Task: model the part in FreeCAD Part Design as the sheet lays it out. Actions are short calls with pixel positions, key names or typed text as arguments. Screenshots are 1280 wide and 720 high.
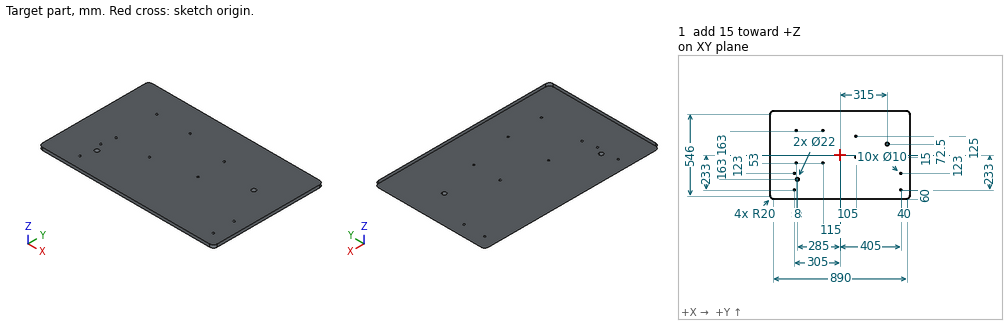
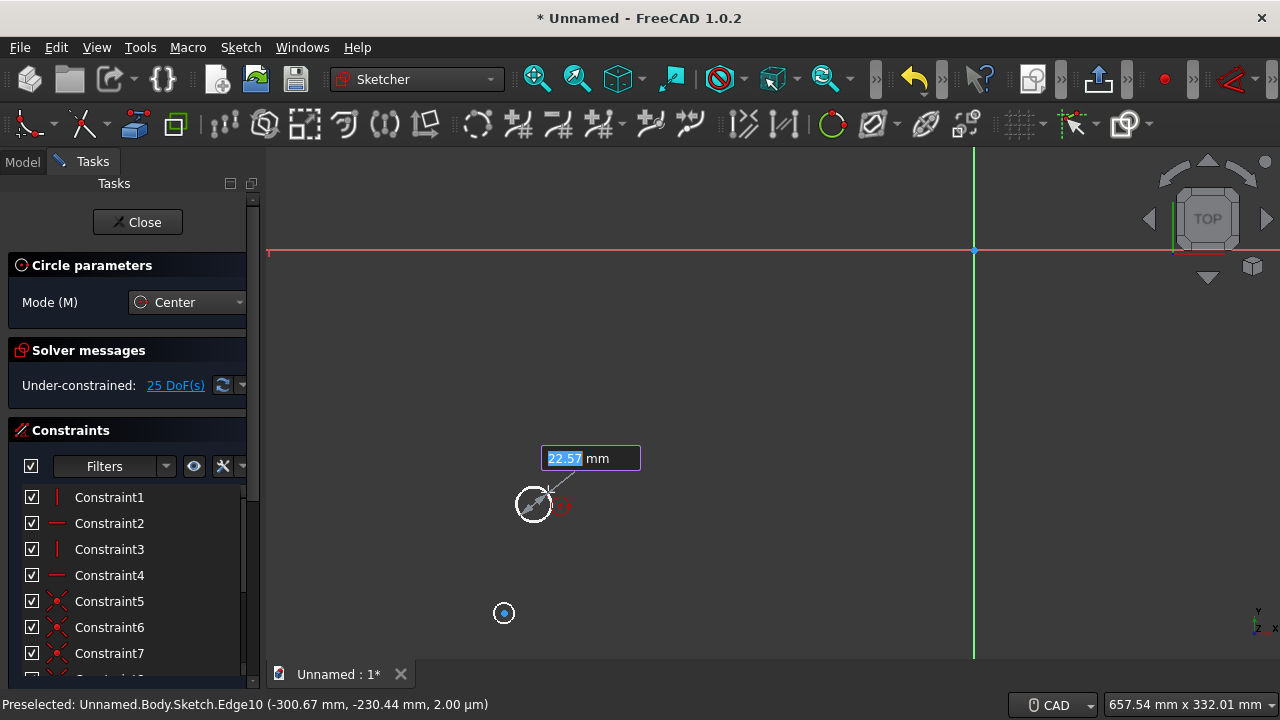
click(547, 489)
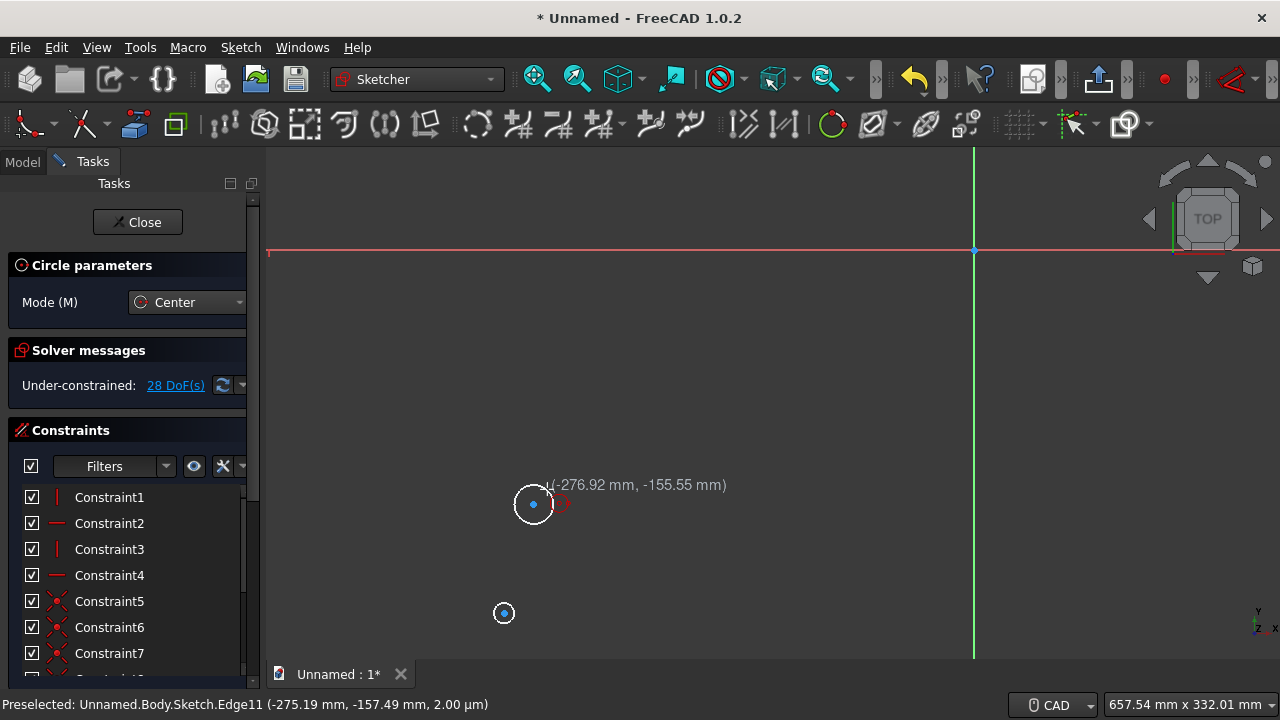
scroll(797, 332, up, 6)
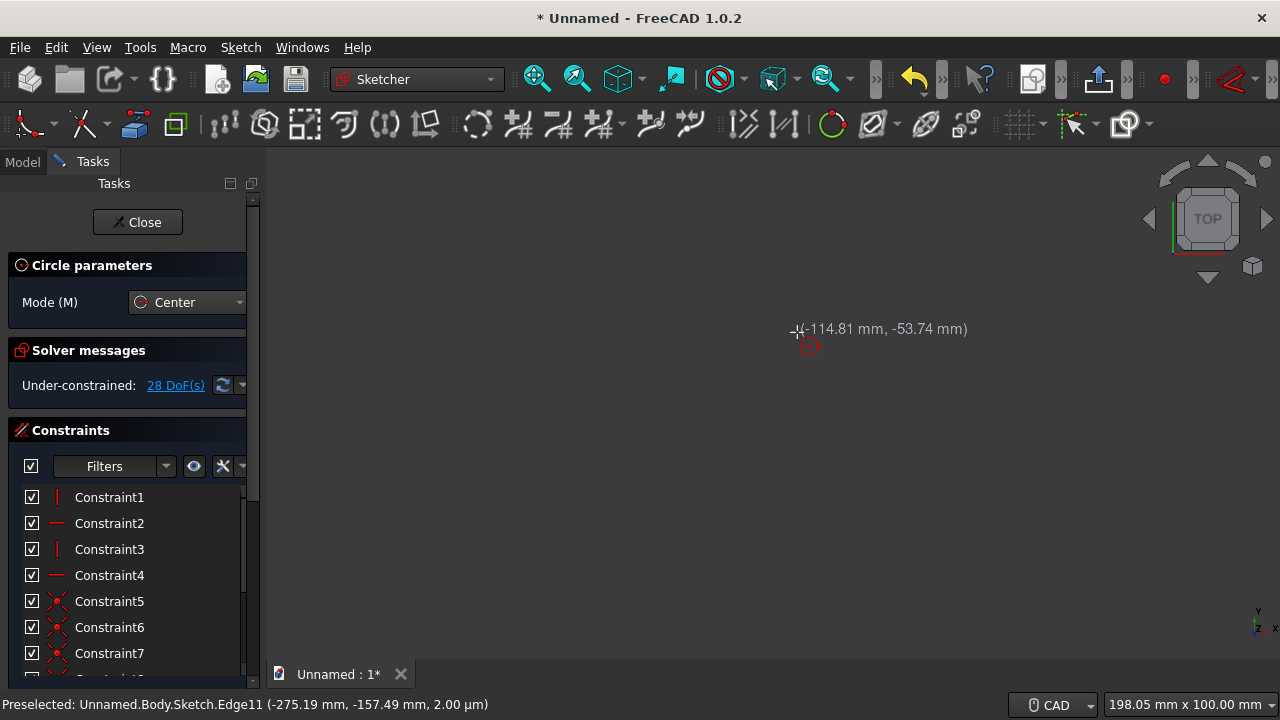
scroll(620, 446, down, 11)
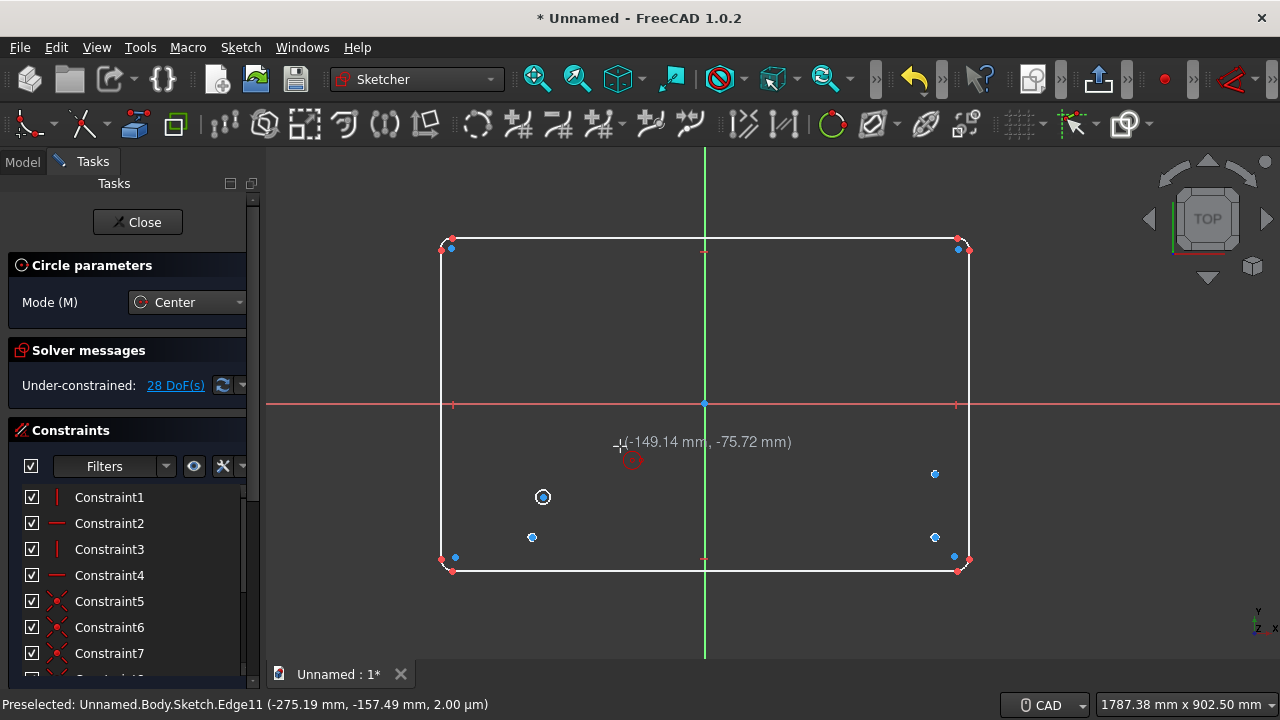
click(640, 434)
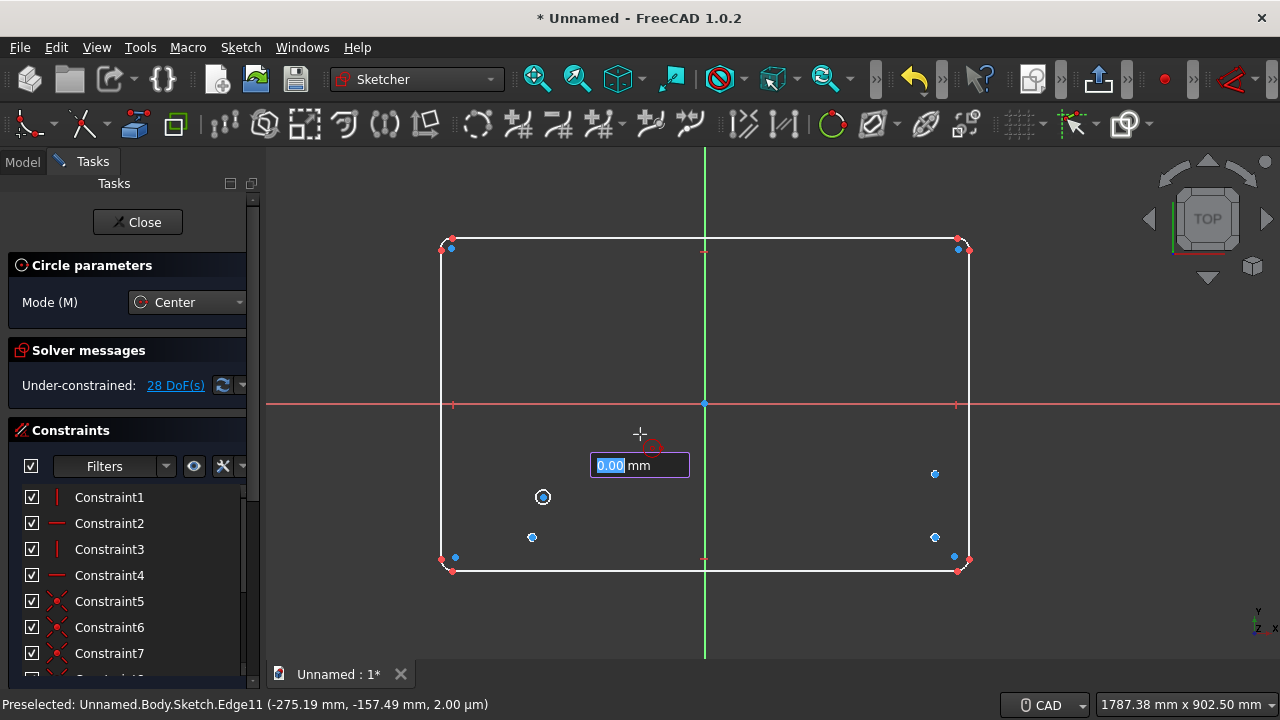
scroll(642, 432, up, 9)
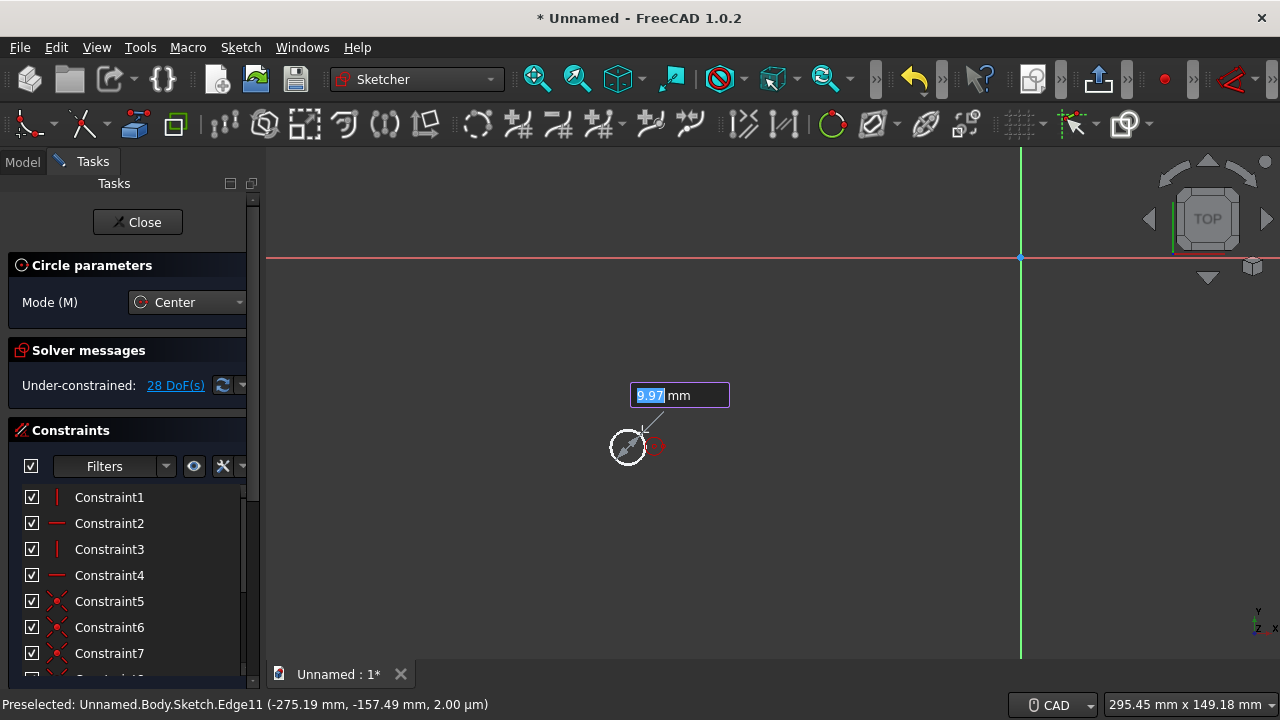
click(638, 428)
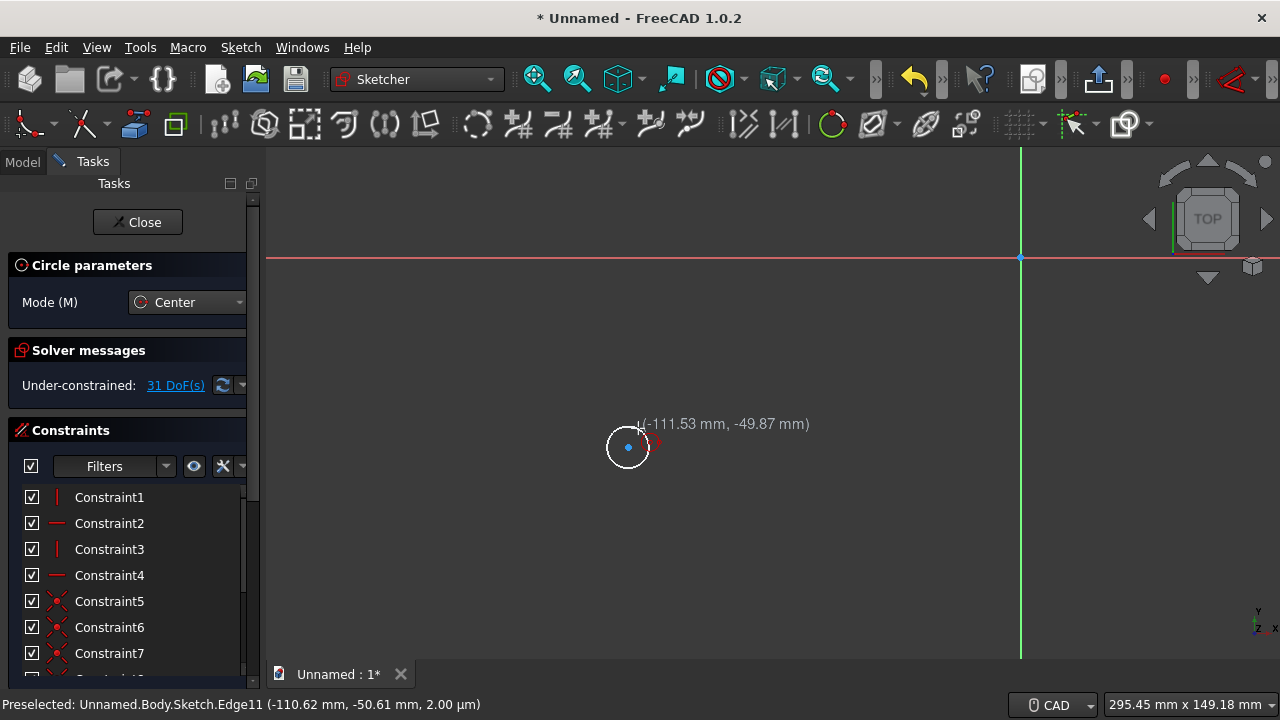
scroll(642, 432, down, 9)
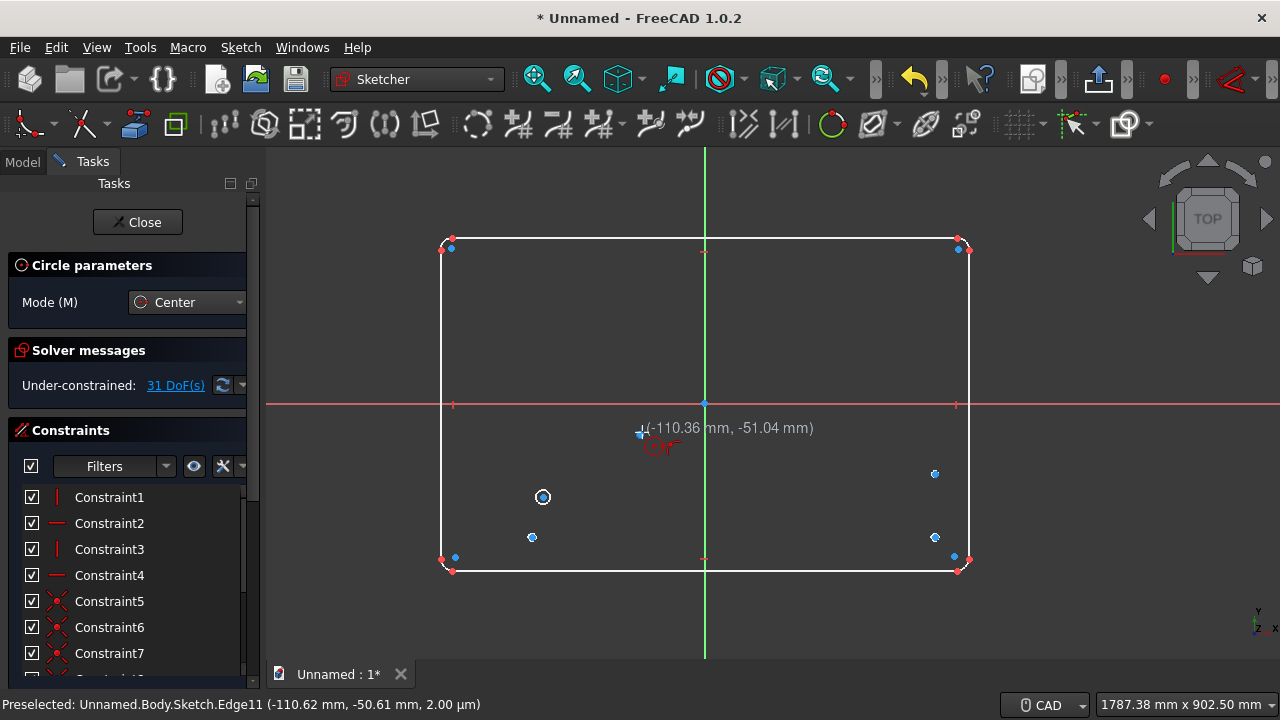
scroll(532, 473, up, 11)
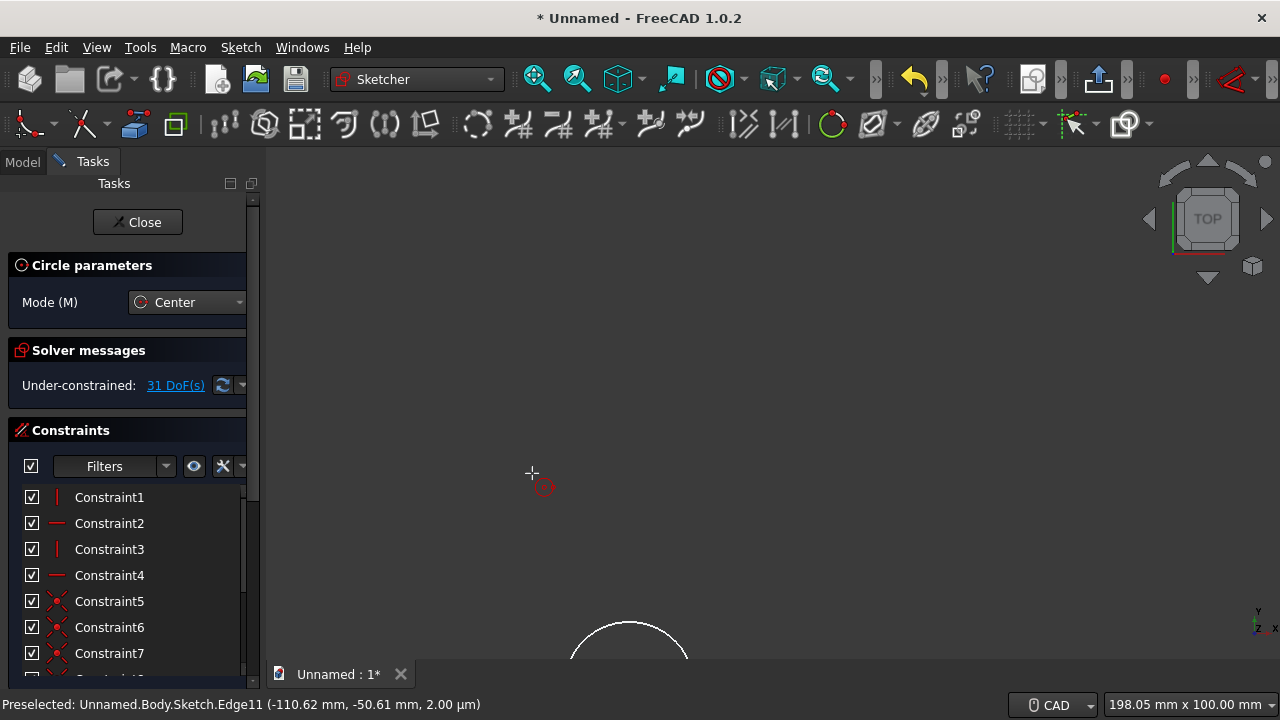
scroll(532, 473, down, 11)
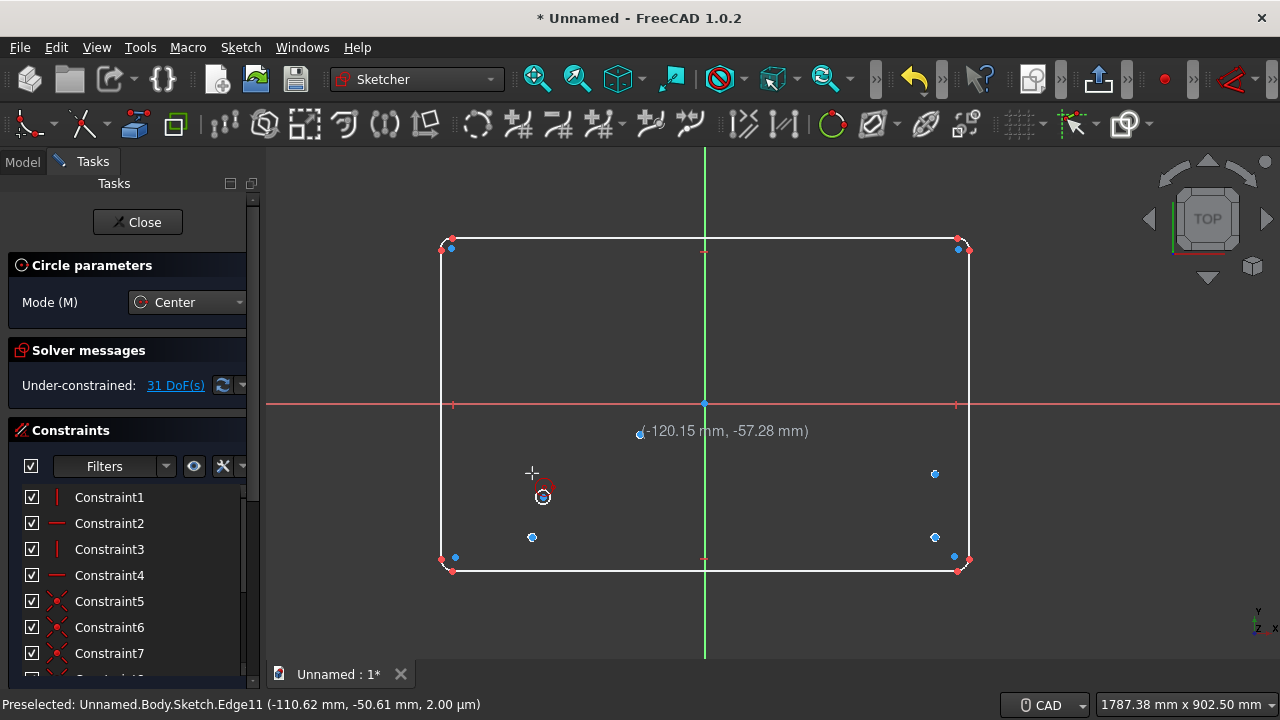
click(532, 473)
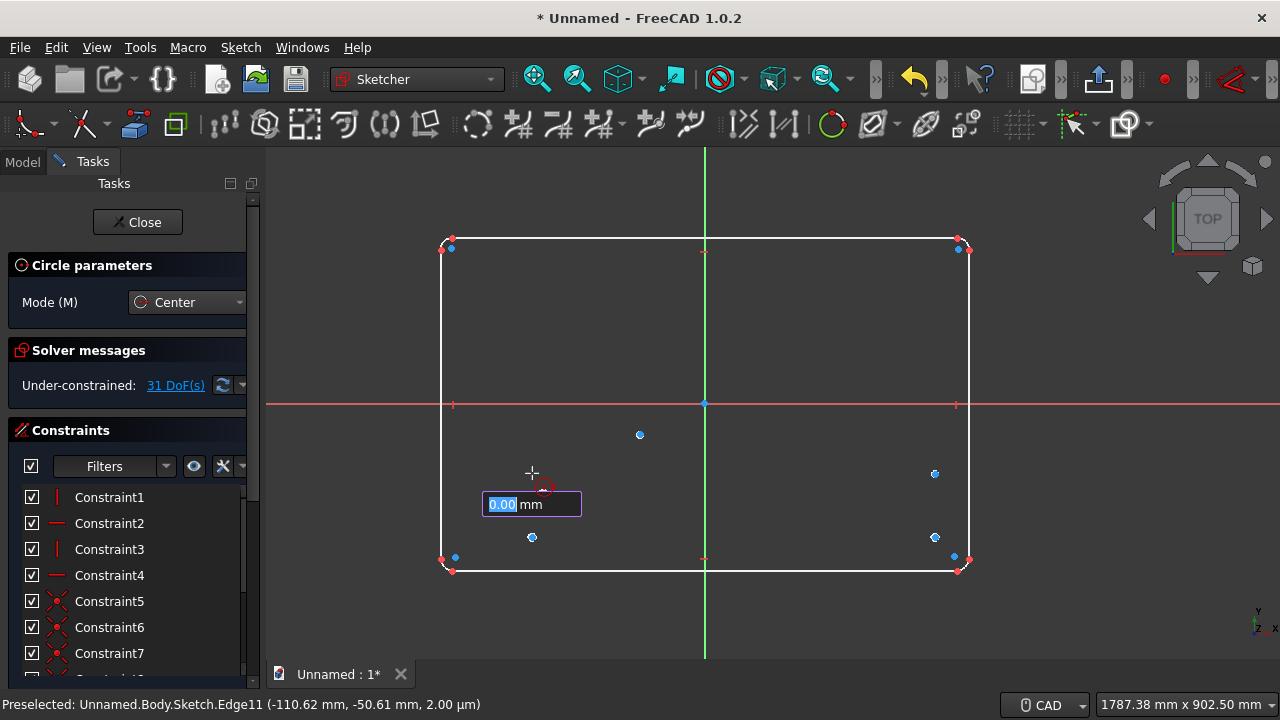
scroll(534, 471, up, 9)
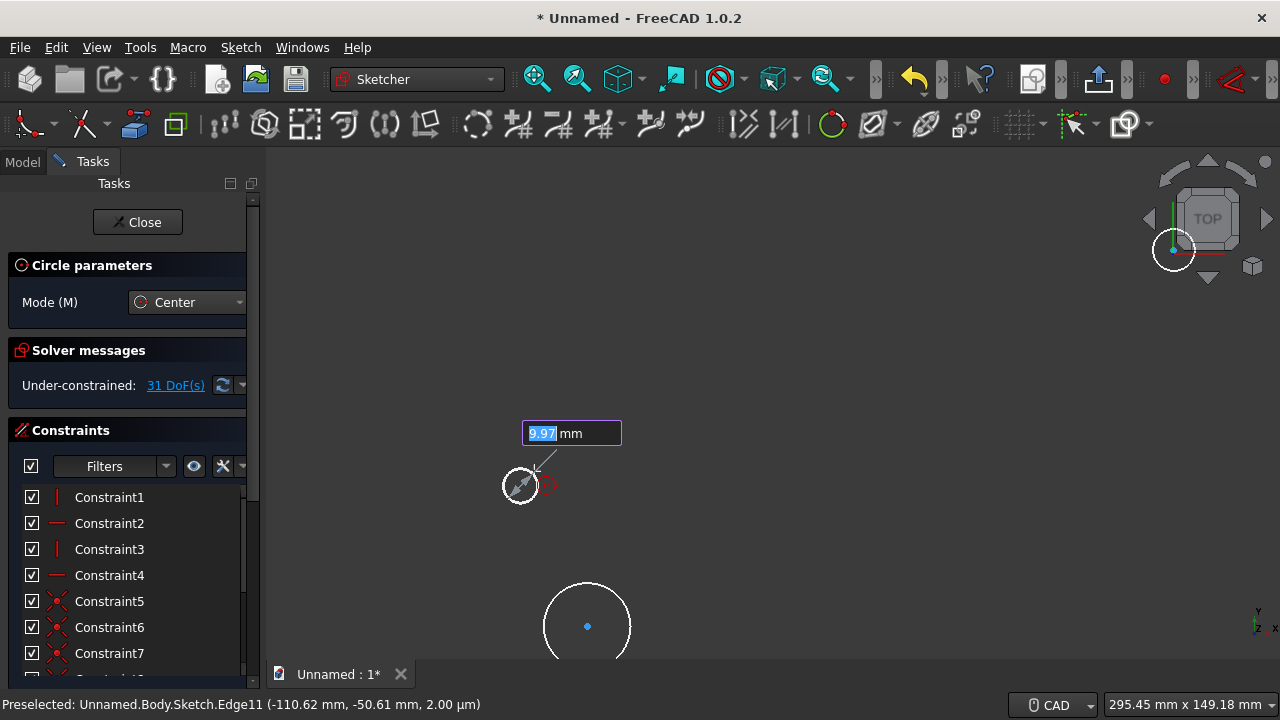
click(532, 471)